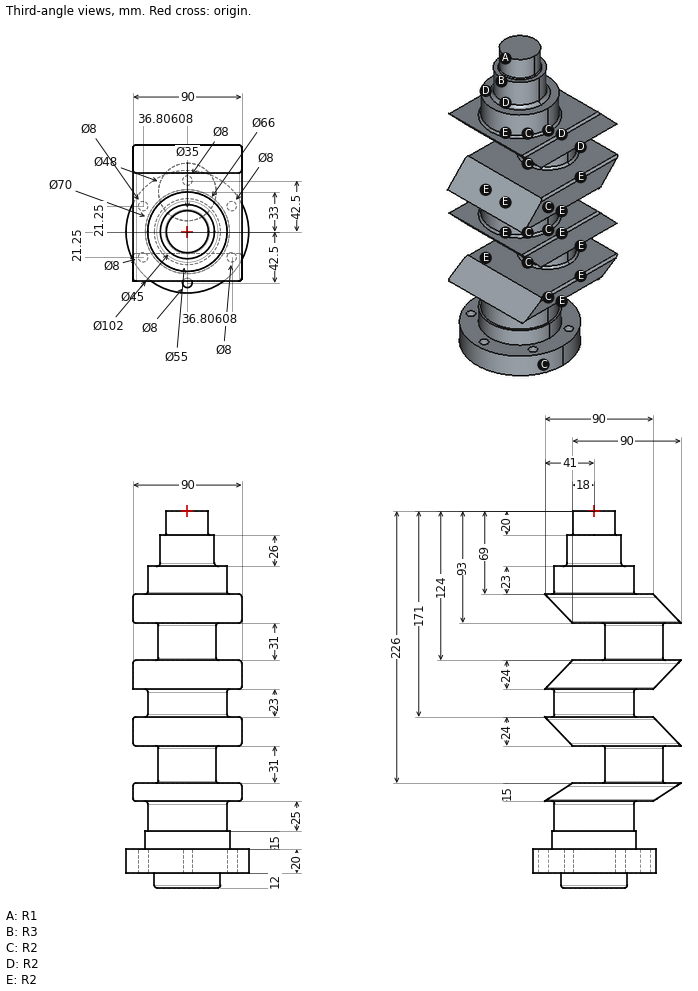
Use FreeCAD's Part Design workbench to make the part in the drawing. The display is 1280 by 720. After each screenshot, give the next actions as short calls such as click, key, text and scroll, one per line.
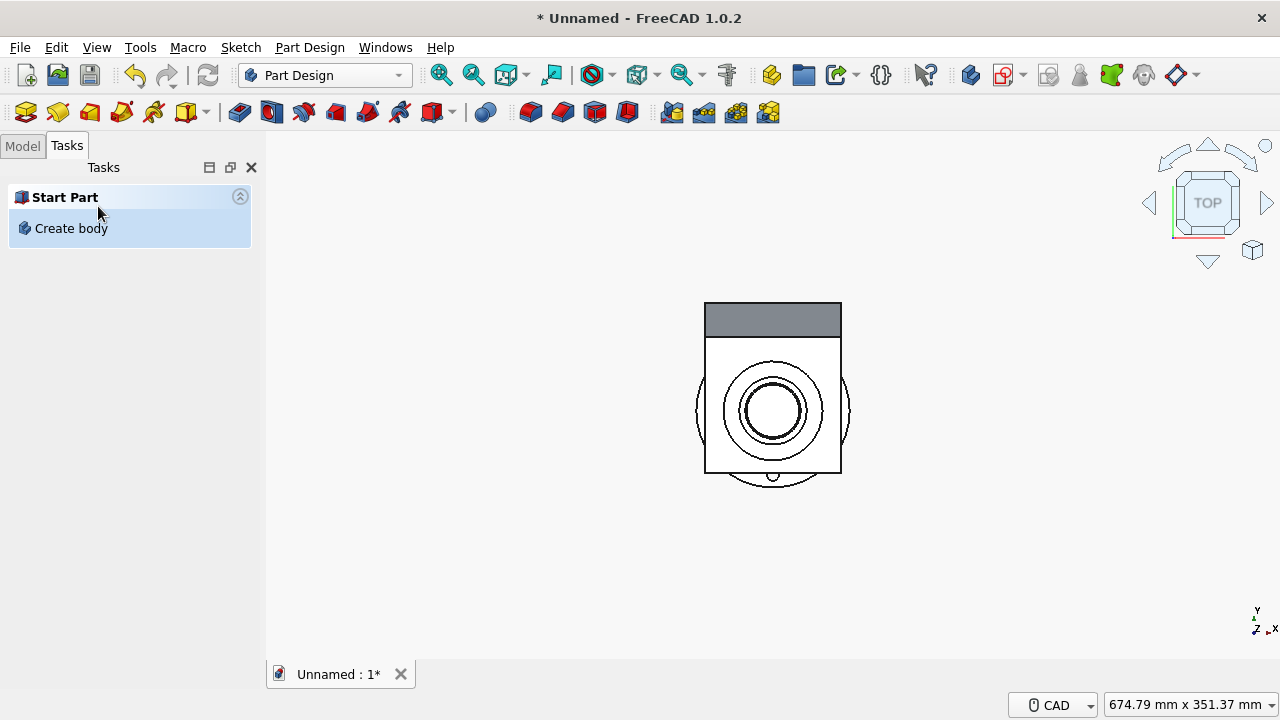
click(442, 76)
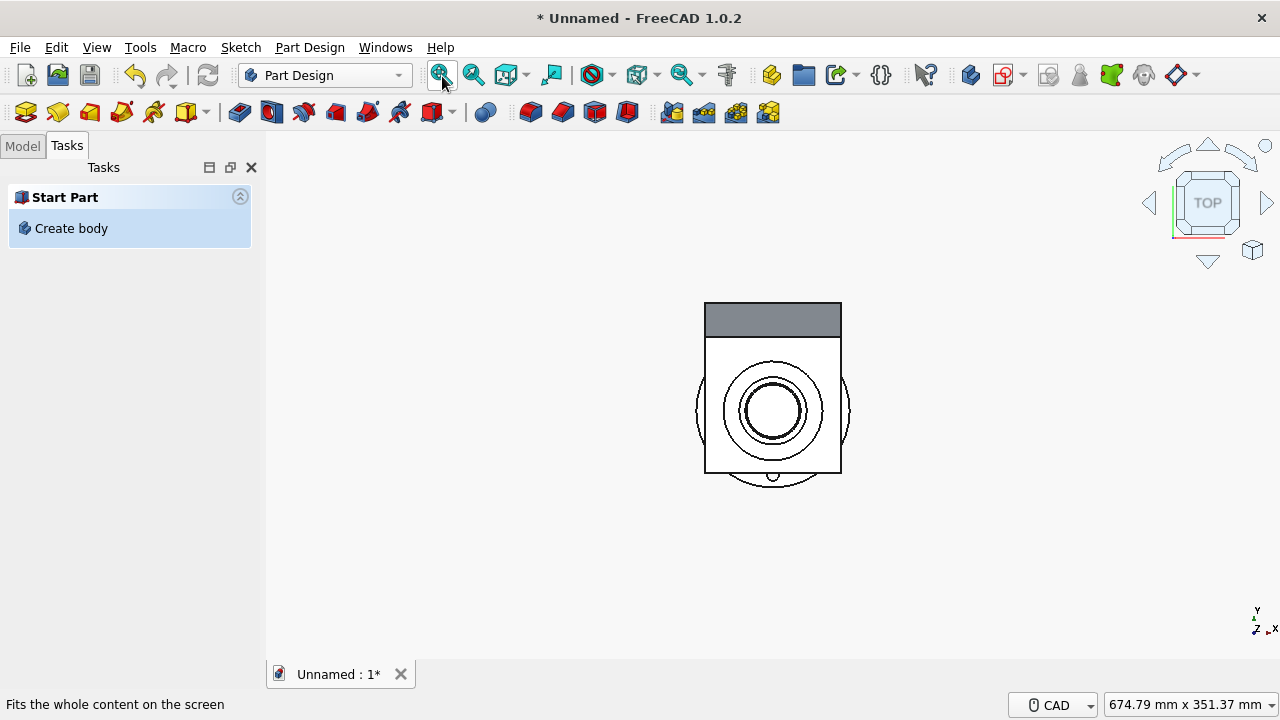
key(0)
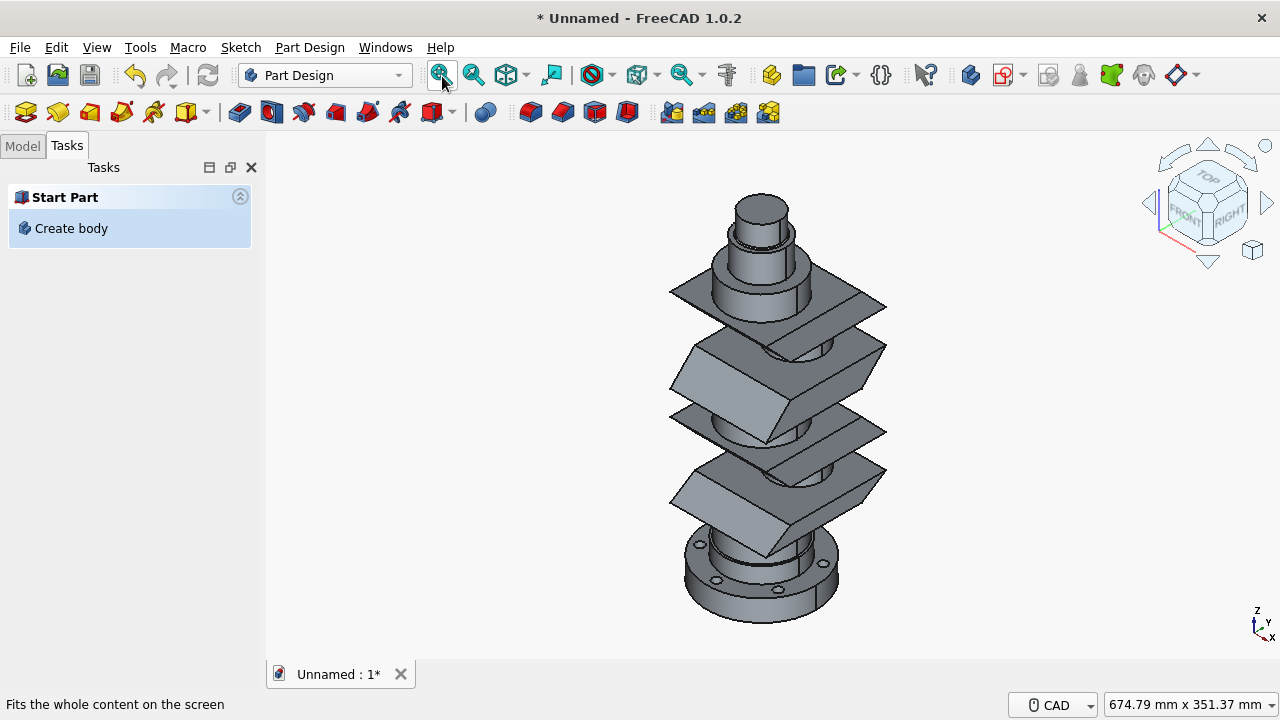
key(1)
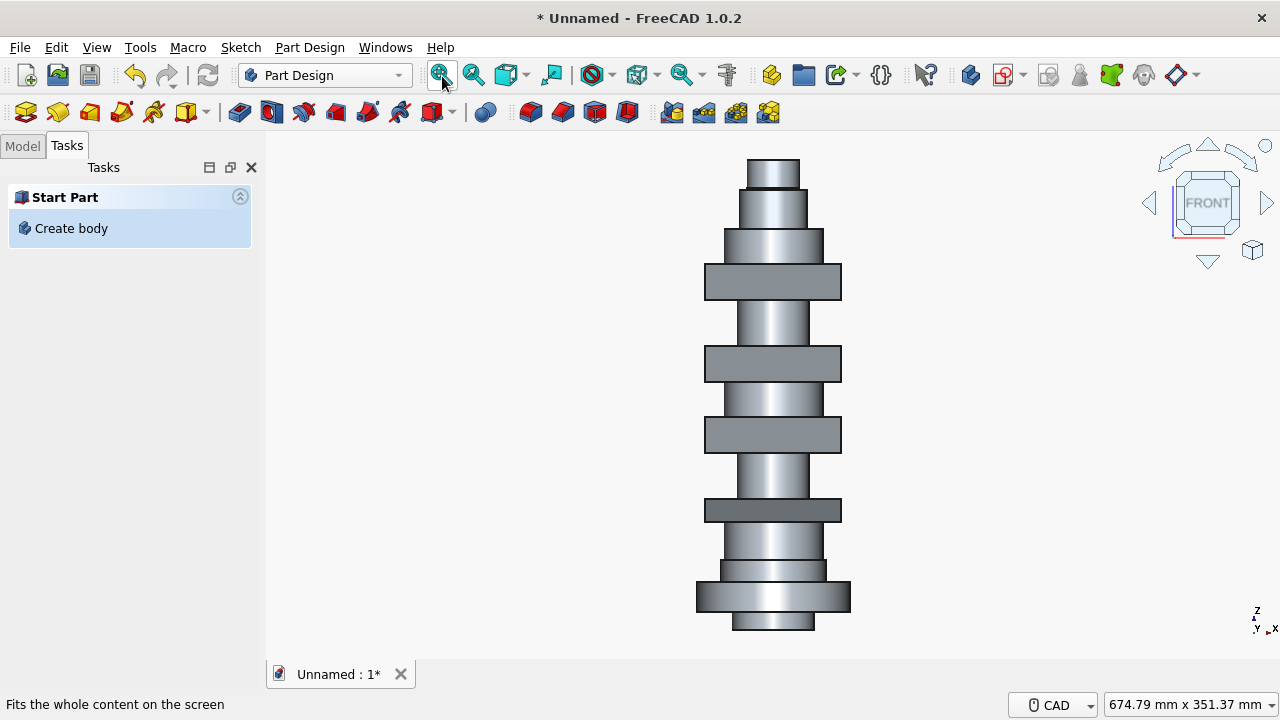
key(3)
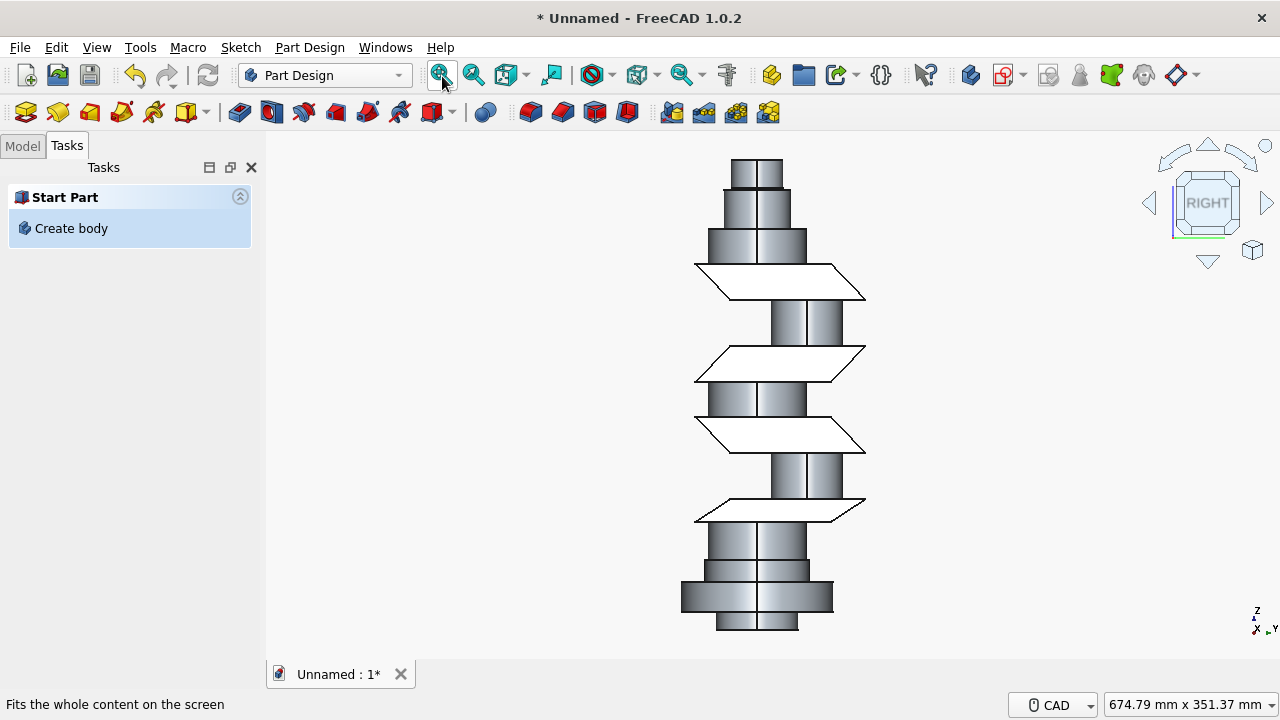
key(5)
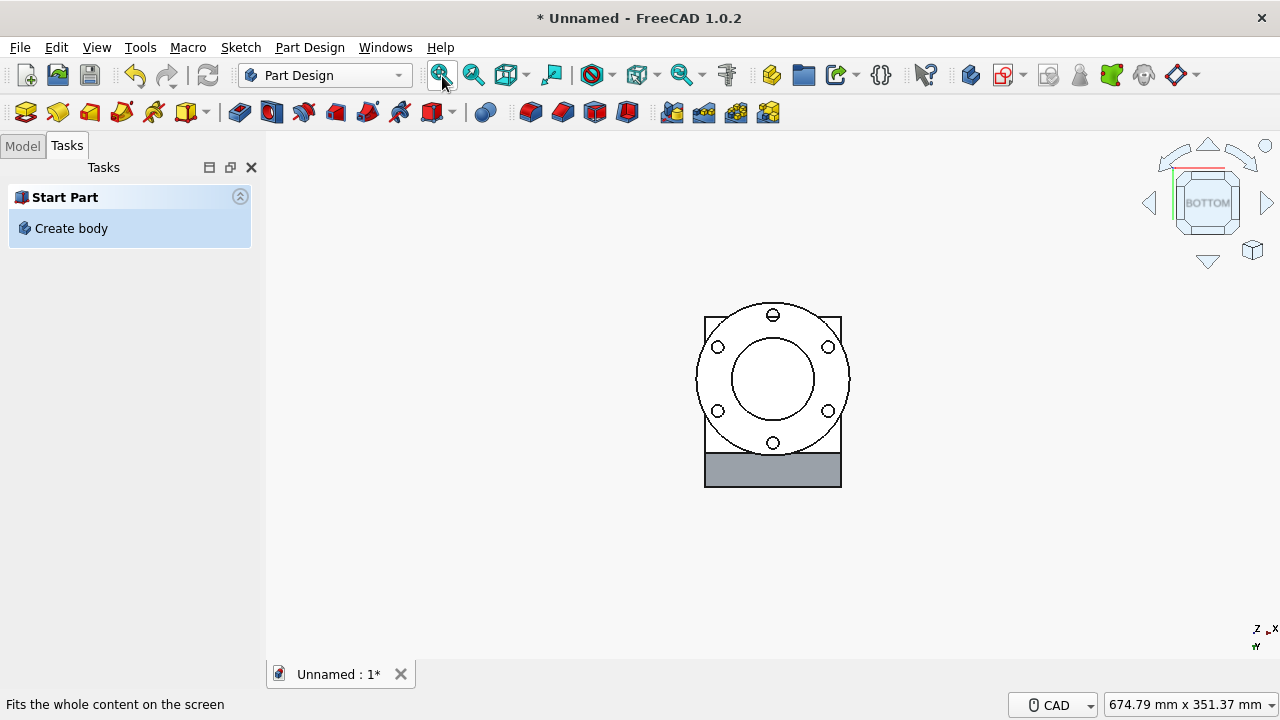
click(442, 76)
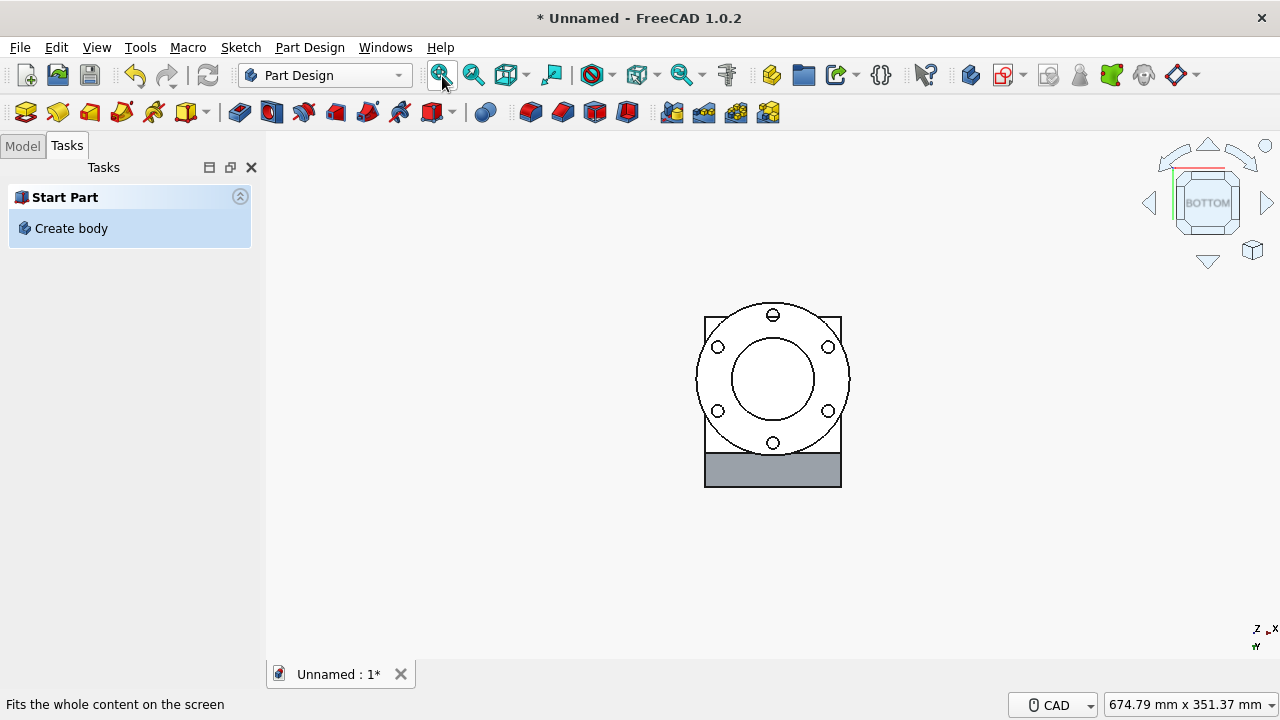
key(4)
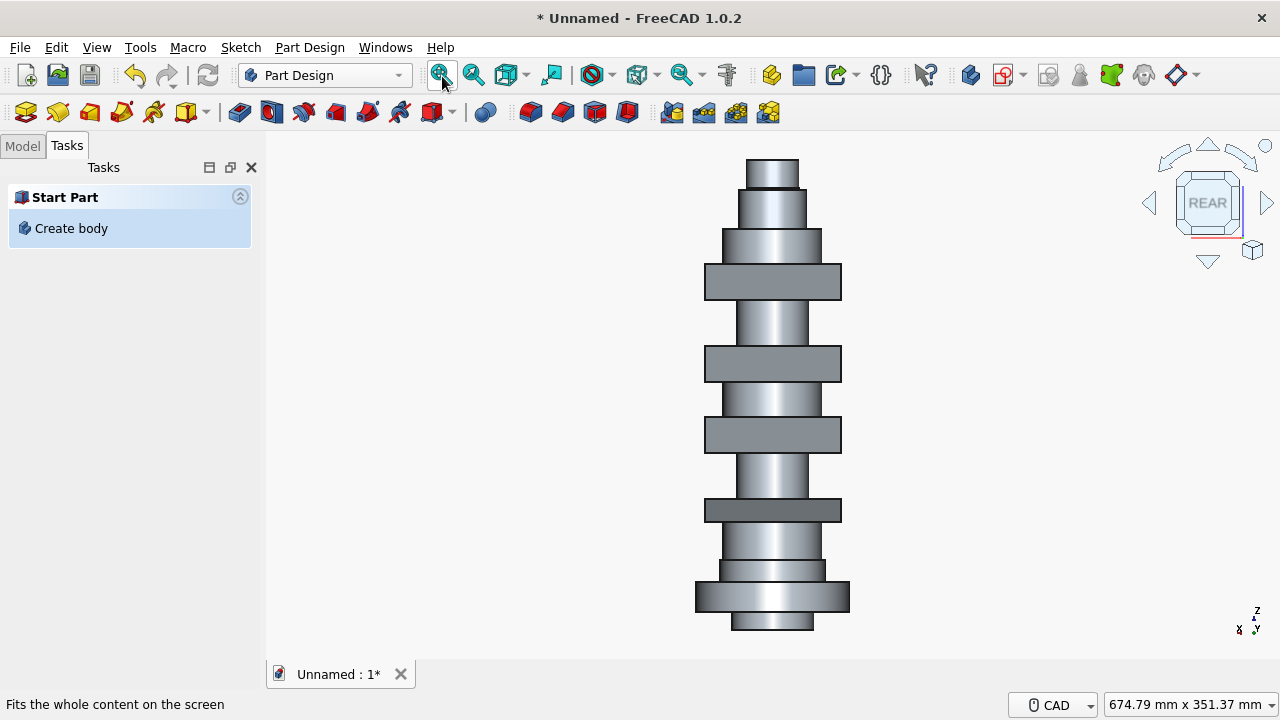
key(6)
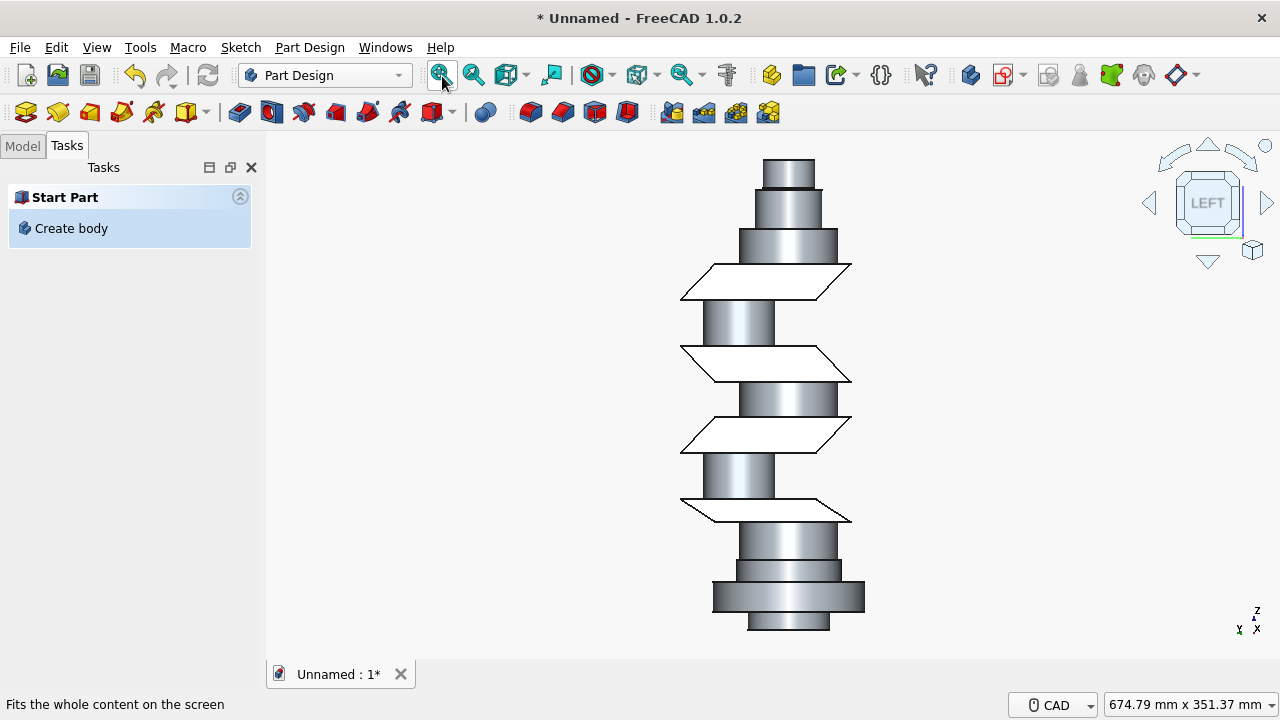
key(v)
key(3)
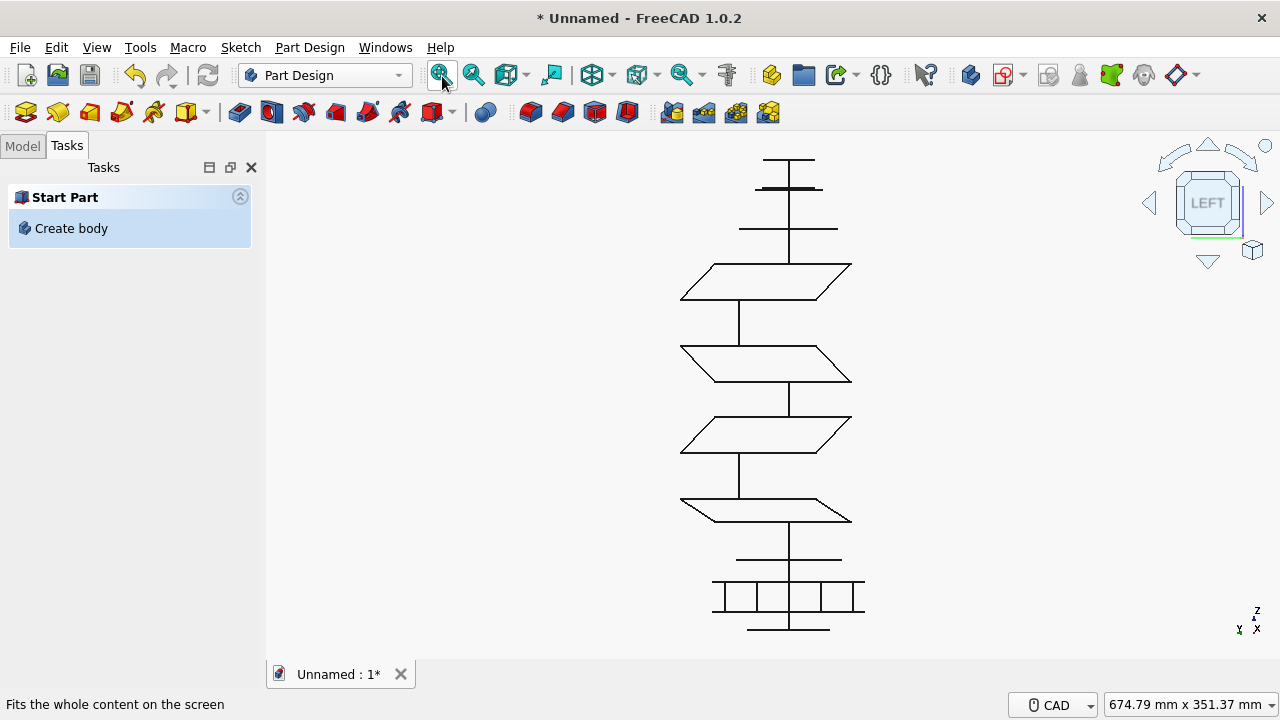
key(0)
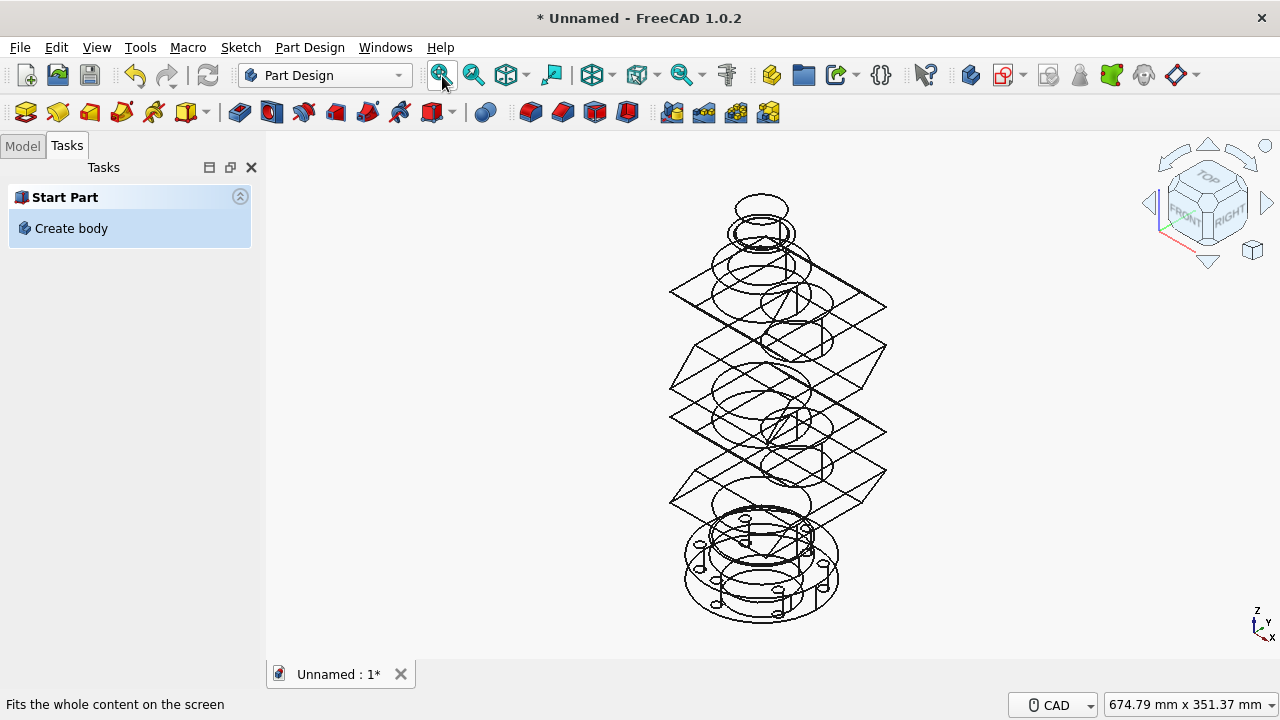
click(728, 262)